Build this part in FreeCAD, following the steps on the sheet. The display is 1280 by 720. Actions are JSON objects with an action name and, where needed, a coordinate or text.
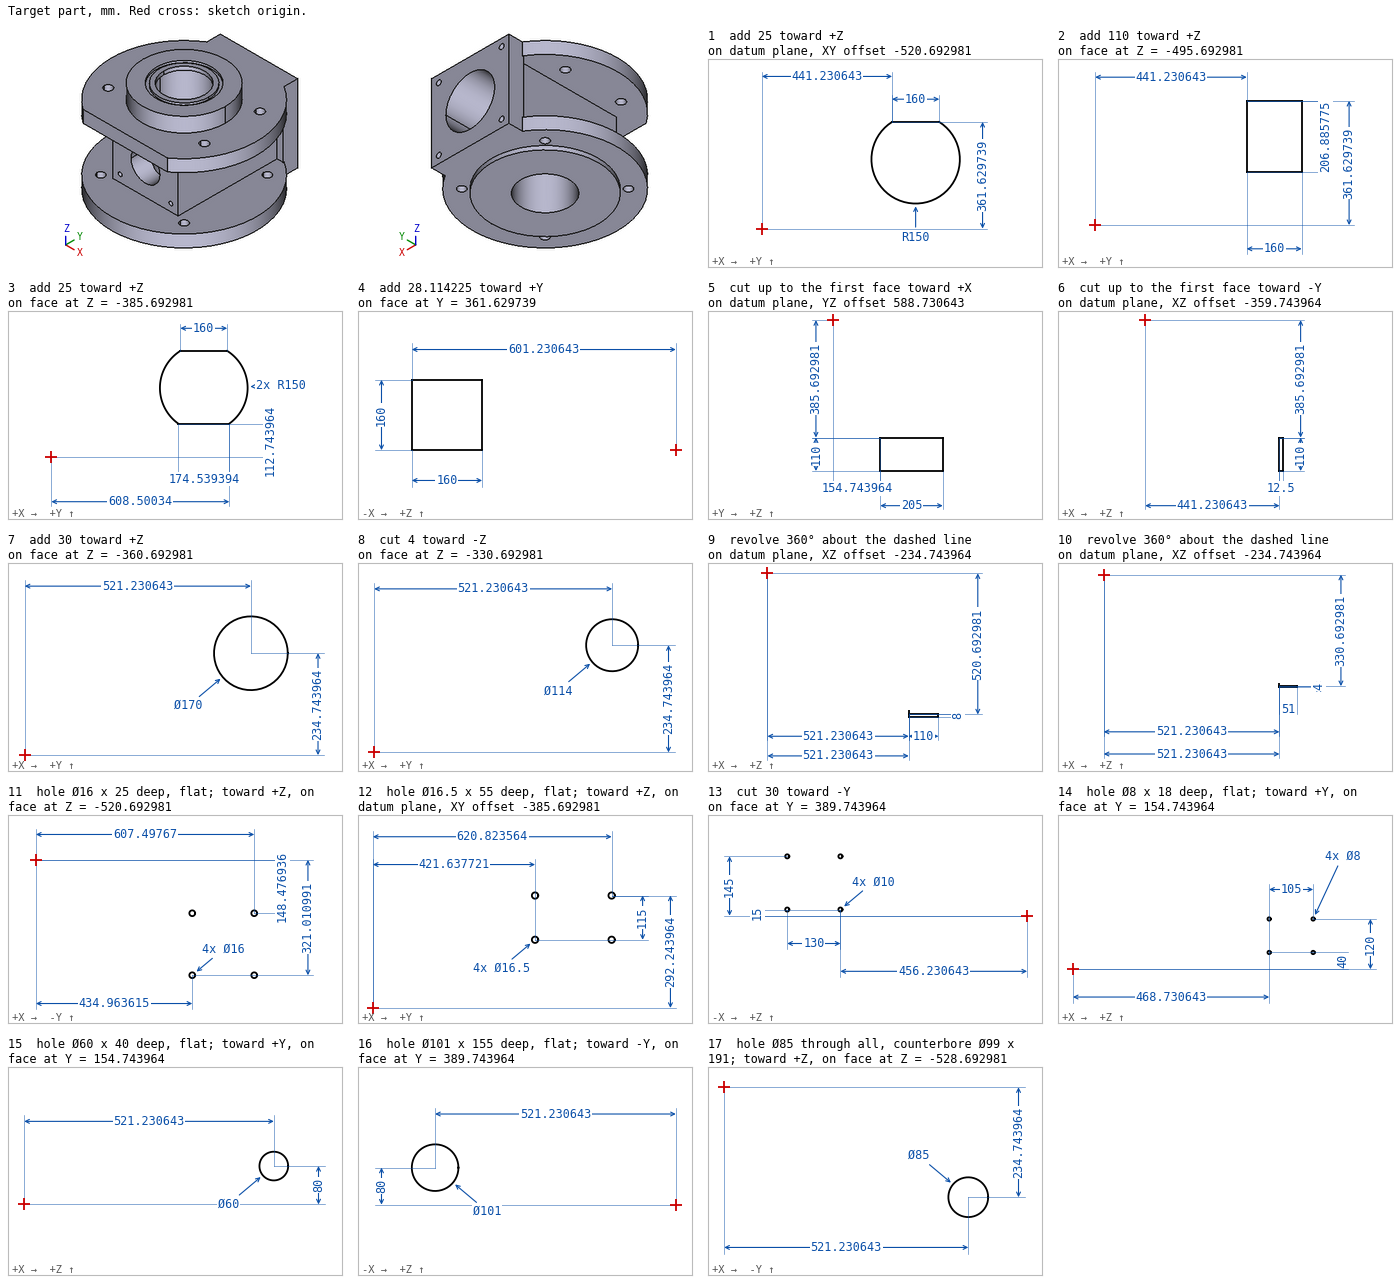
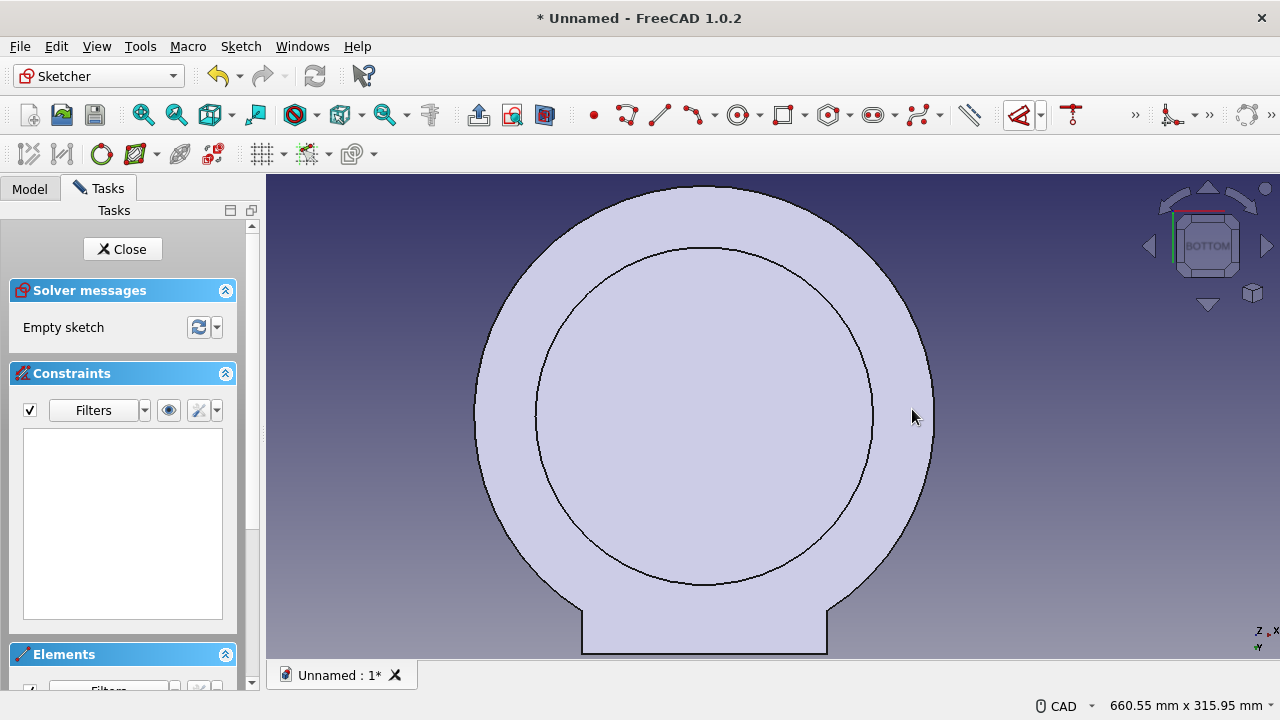
{"action": "left_click", "coordinate": [738, 116]}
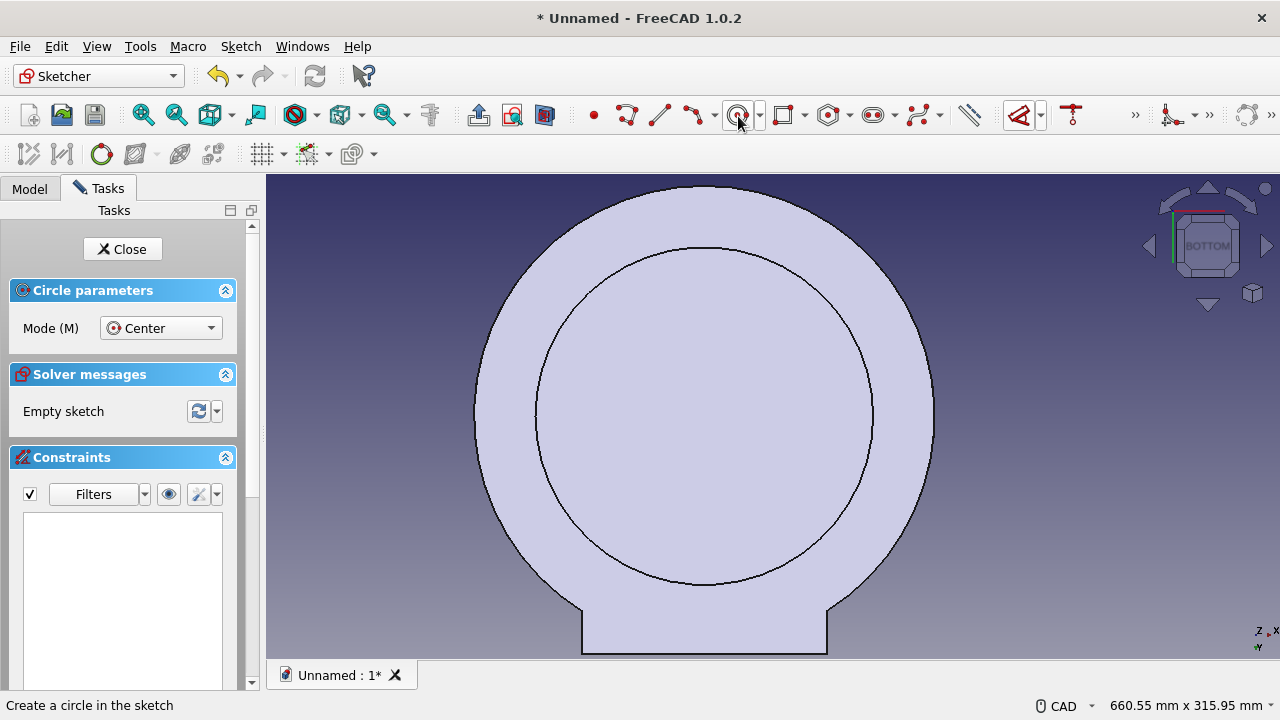
{"action": "scroll", "coordinate": [572, 549], "scroll_direction": "up", "scroll_amount": 4}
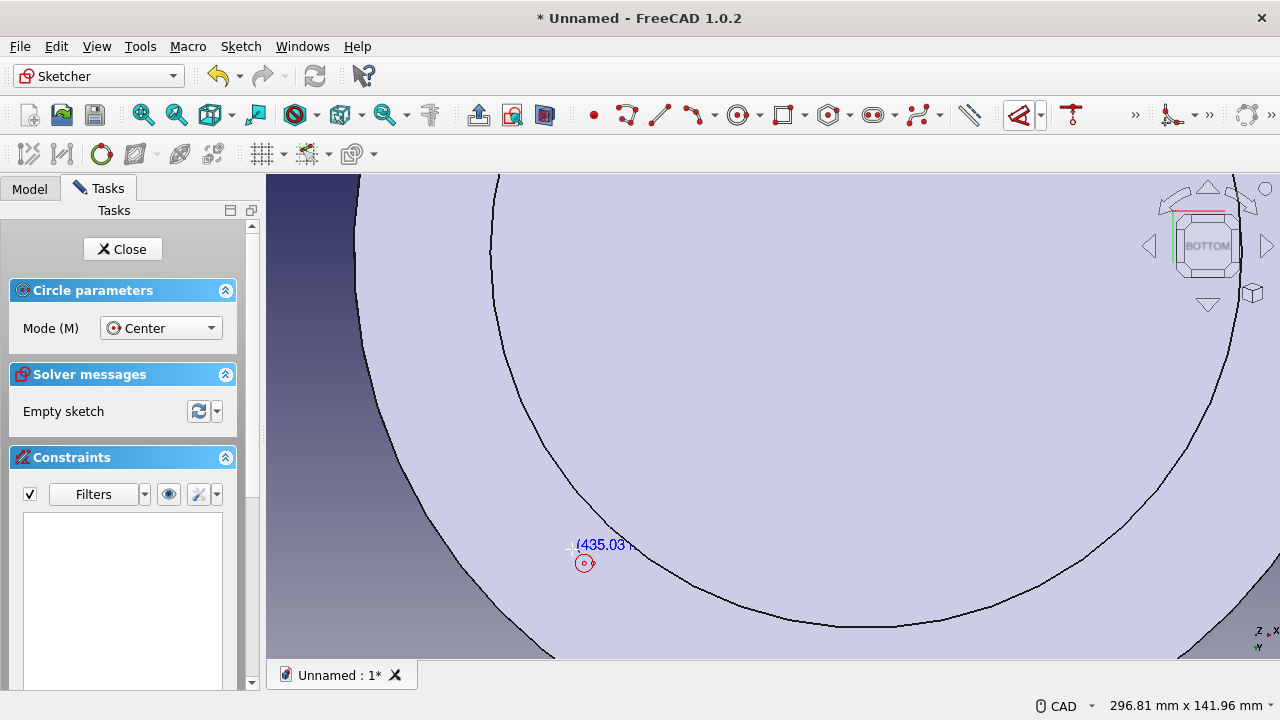
{"action": "left_click", "coordinate": [571, 547]}
{"action": "left_click", "coordinate": [591, 528]}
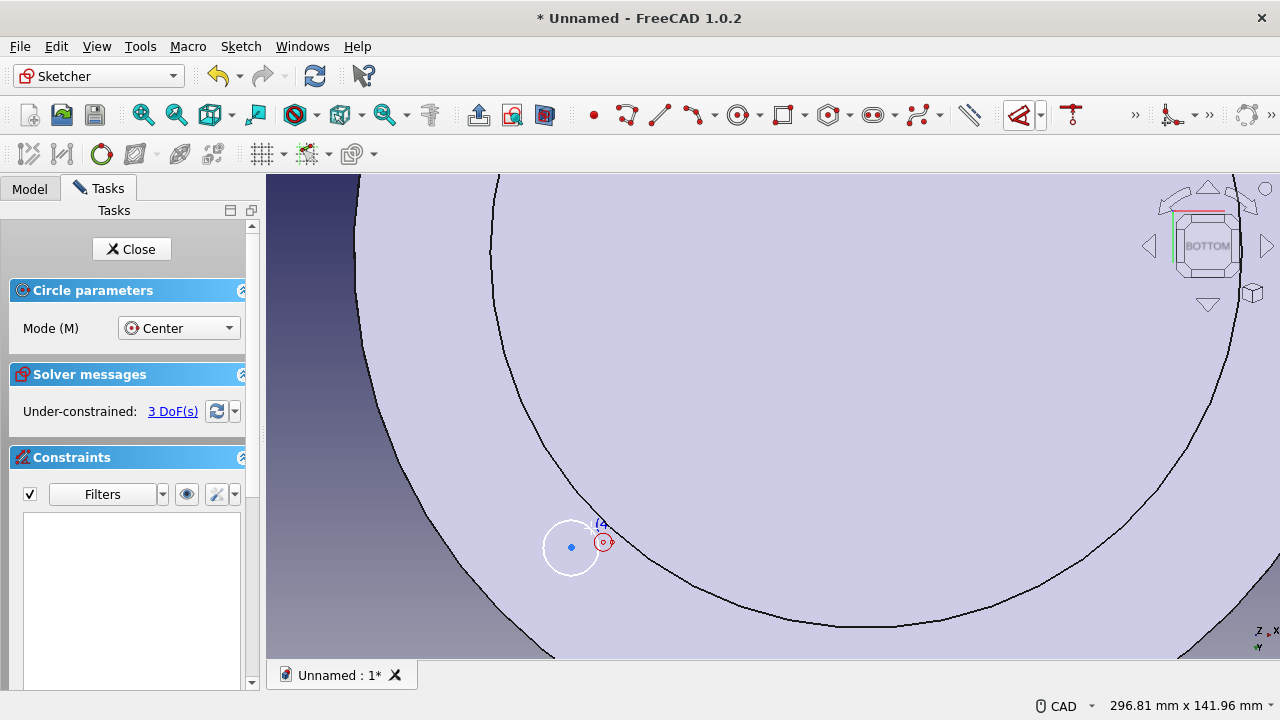
{"action": "scroll", "coordinate": [573, 550], "scroll_direction": "down", "scroll_amount": 4}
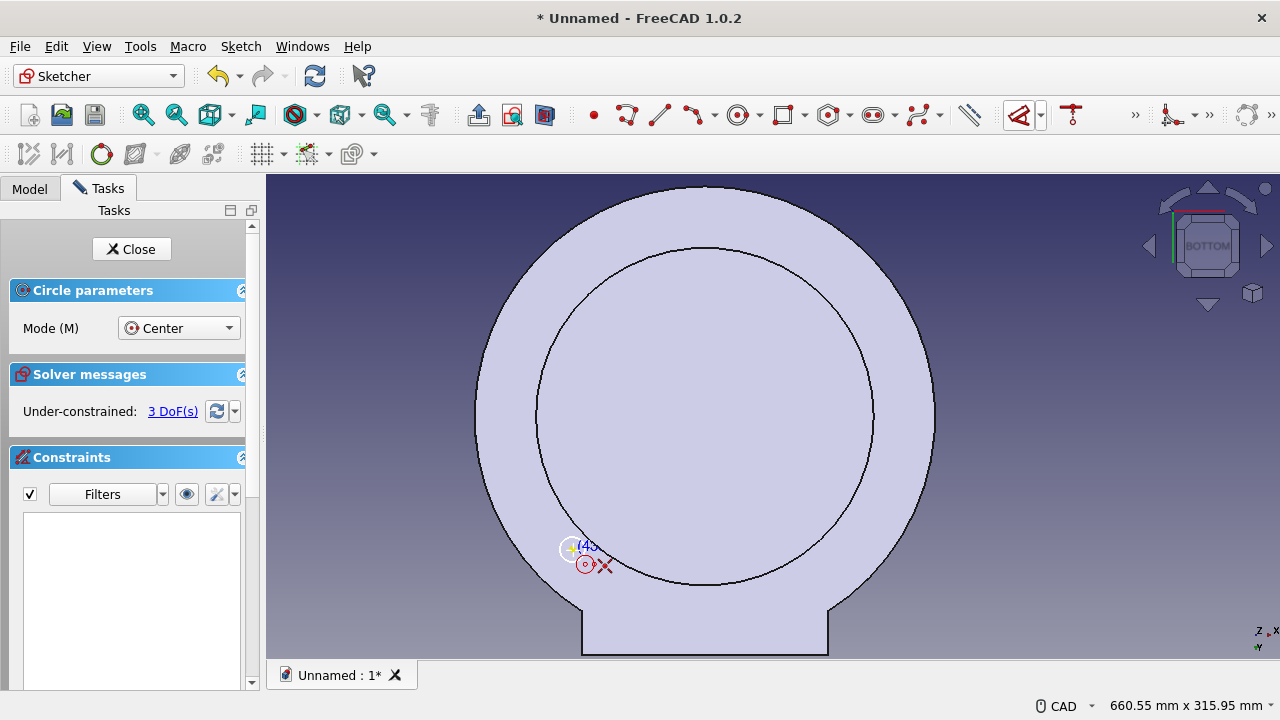
{"action": "scroll", "coordinate": [837, 284], "scroll_direction": "up", "scroll_amount": 4}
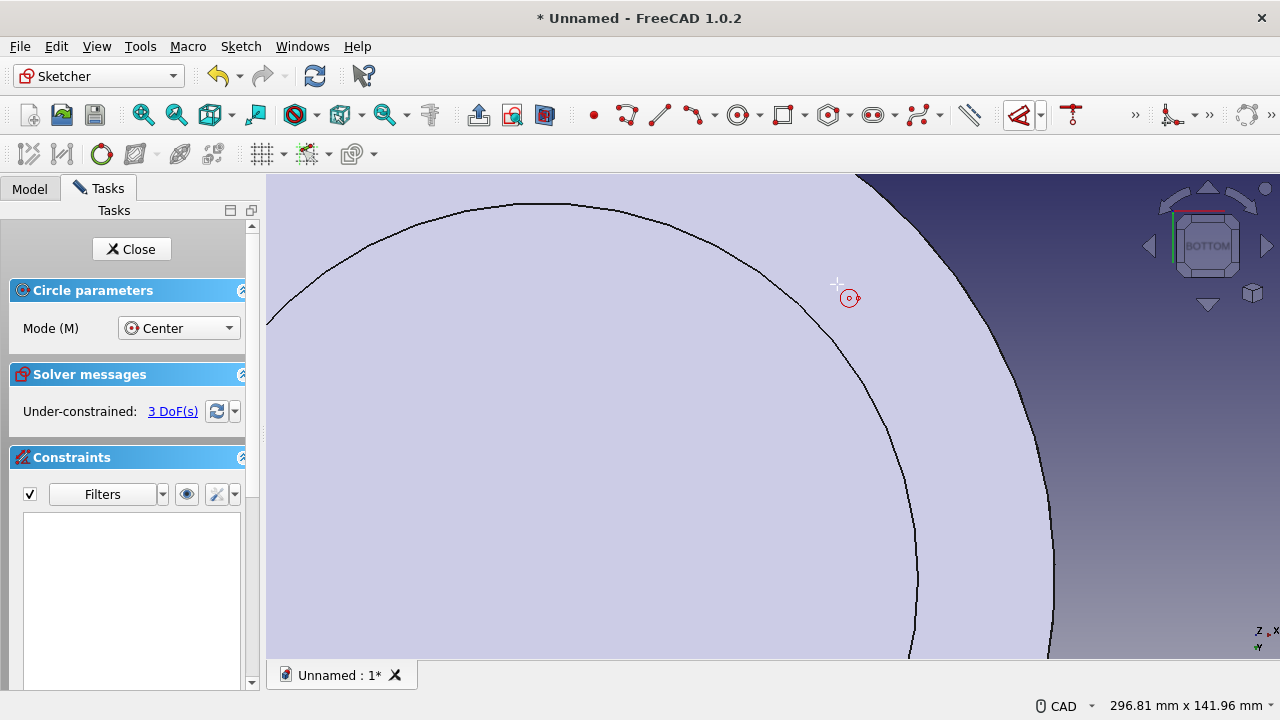
{"action": "left_click", "coordinate": [837, 284]}
{"action": "left_click", "coordinate": [856, 265]}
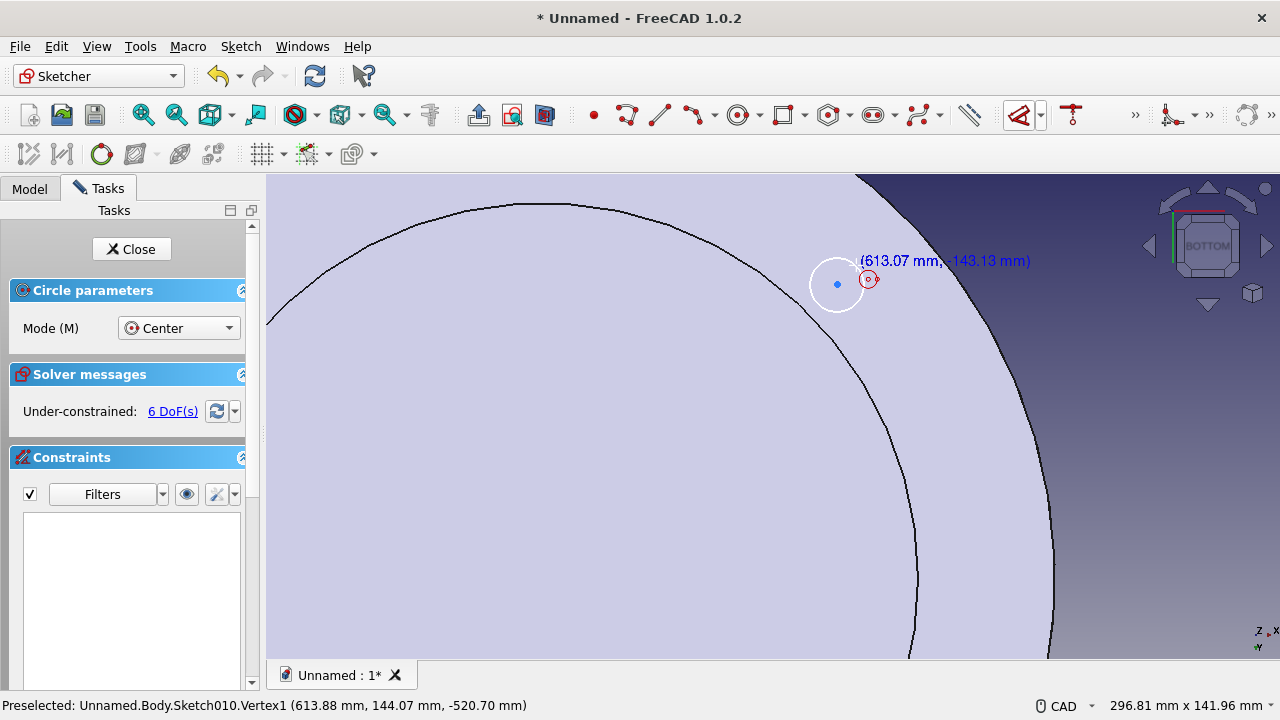
{"action": "scroll", "coordinate": [837, 284], "scroll_direction": "down", "scroll_amount": 4}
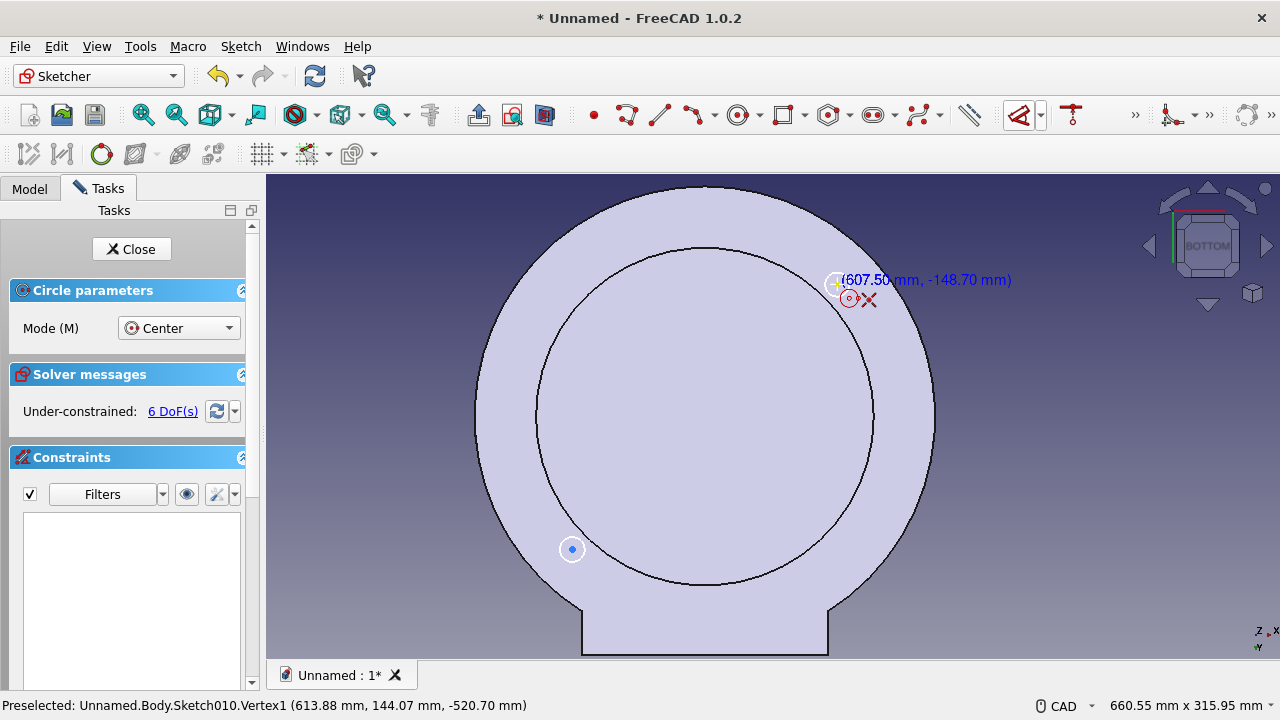
{"action": "scroll", "coordinate": [572, 284], "scroll_direction": "up", "scroll_amount": 4}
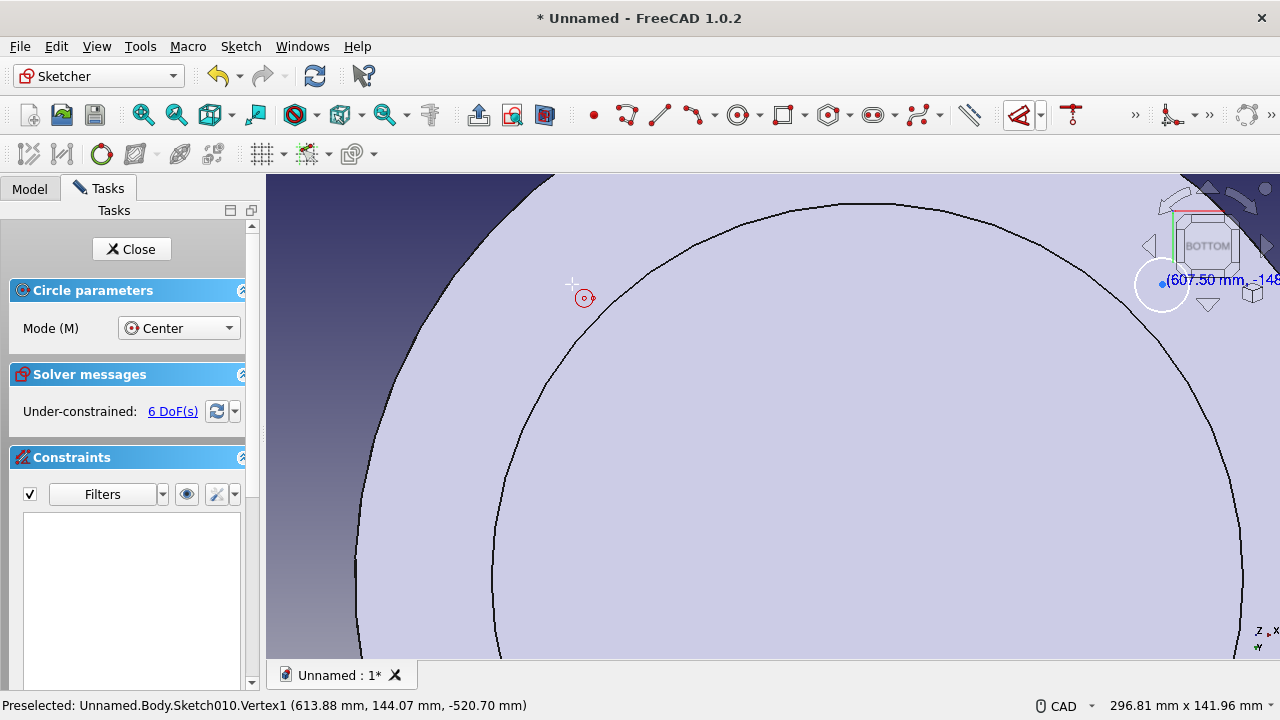
{"action": "left_click", "coordinate": [573, 284]}
{"action": "left_click", "coordinate": [592, 265]}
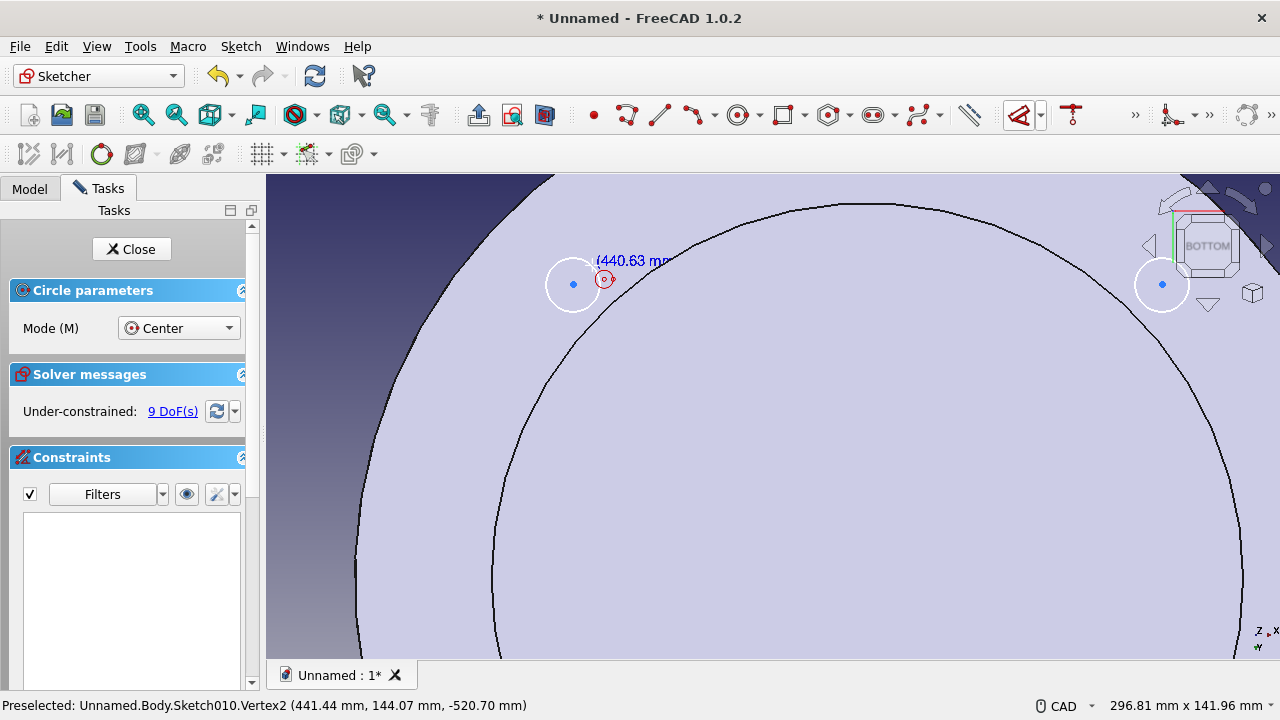
{"action": "scroll", "coordinate": [572, 284], "scroll_direction": "down", "scroll_amount": 4}